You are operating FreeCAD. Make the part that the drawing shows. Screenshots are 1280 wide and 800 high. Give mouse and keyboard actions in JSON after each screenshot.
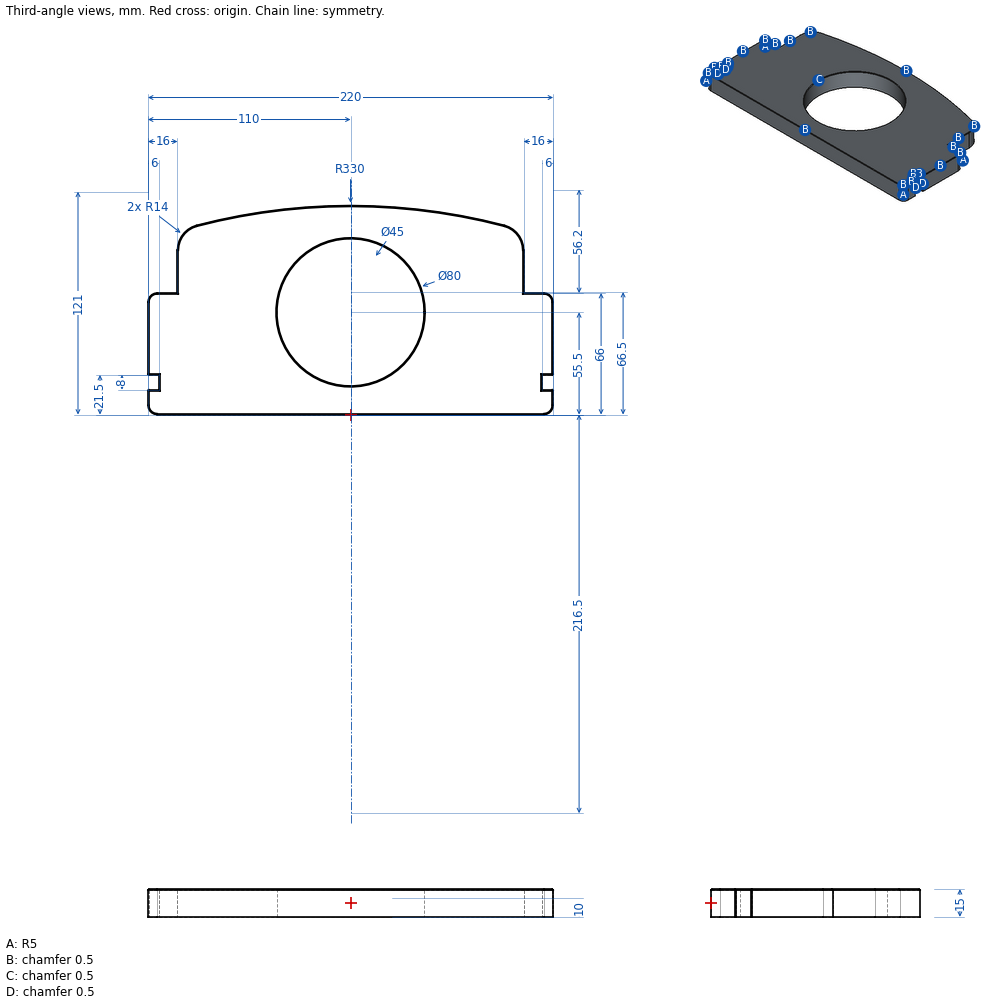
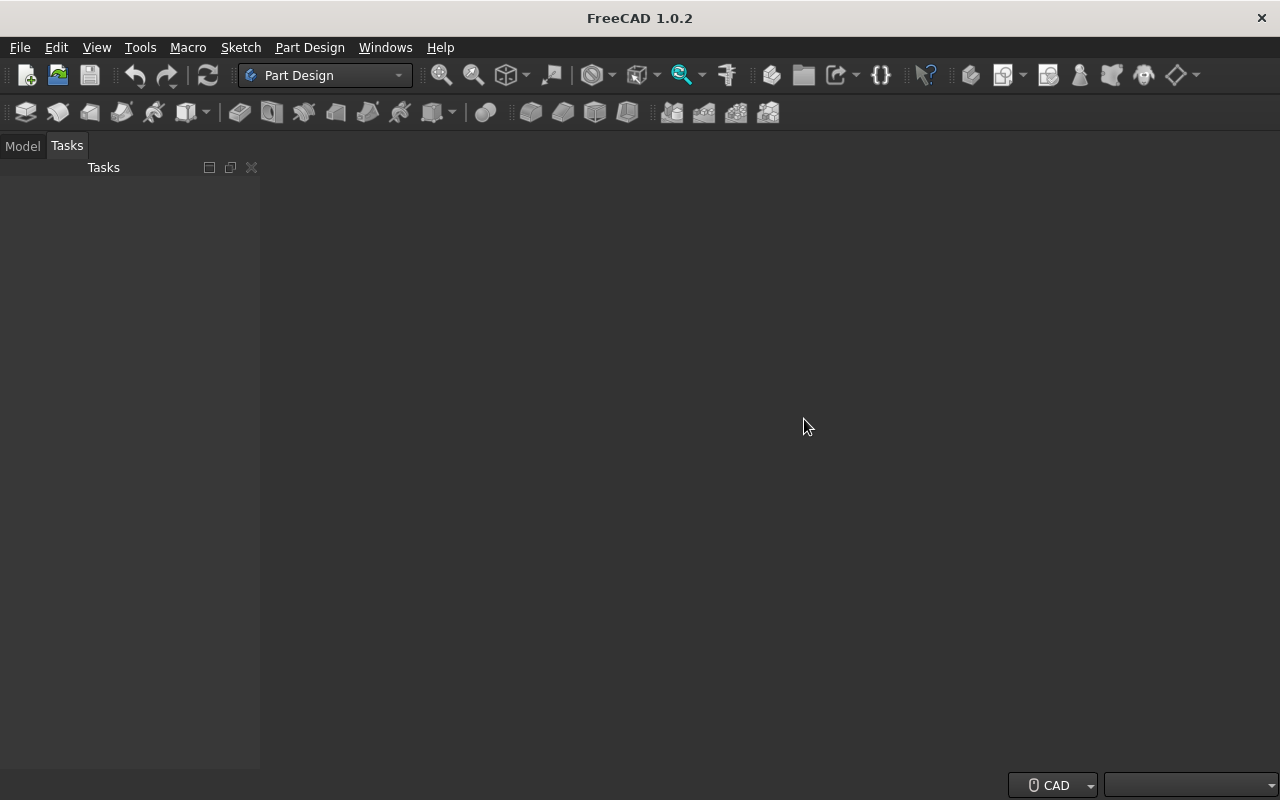
{"action": "left_click", "coordinate": [26, 76]}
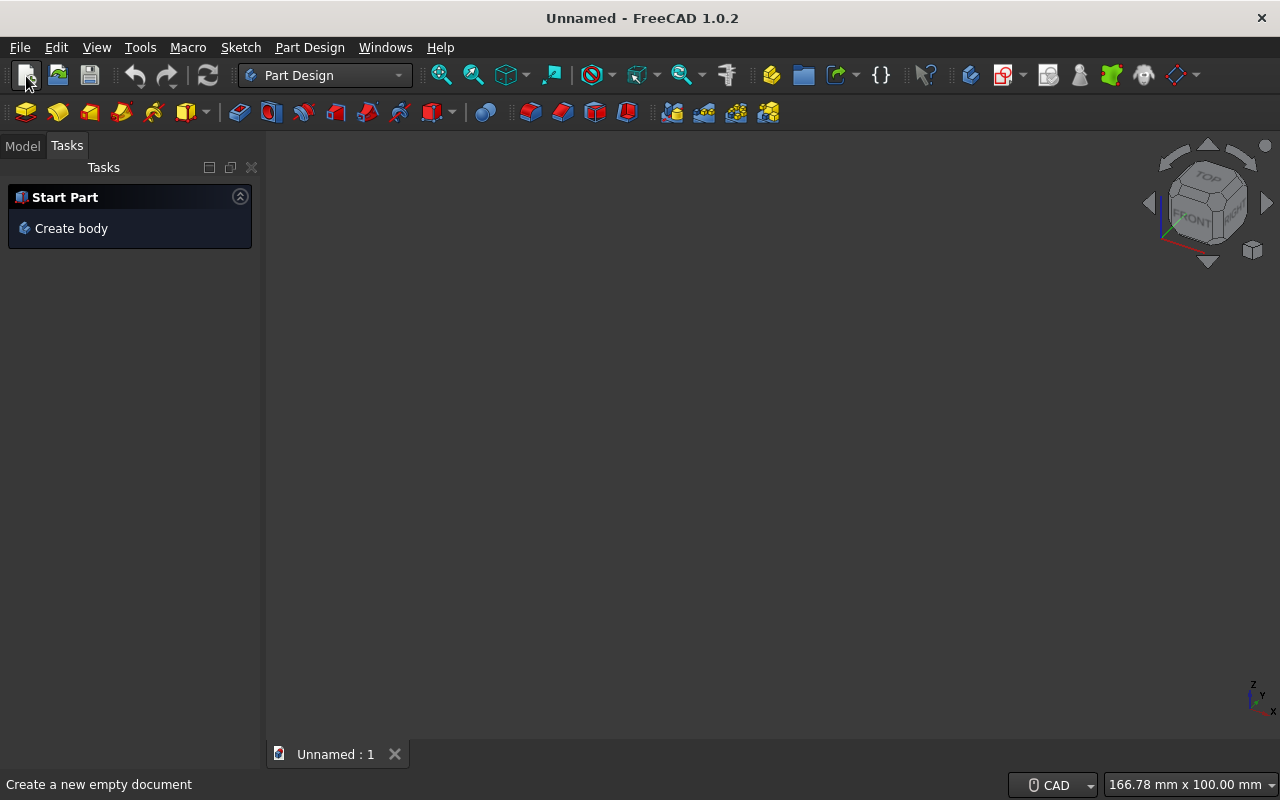
{"action": "left_click", "coordinate": [1004, 76]}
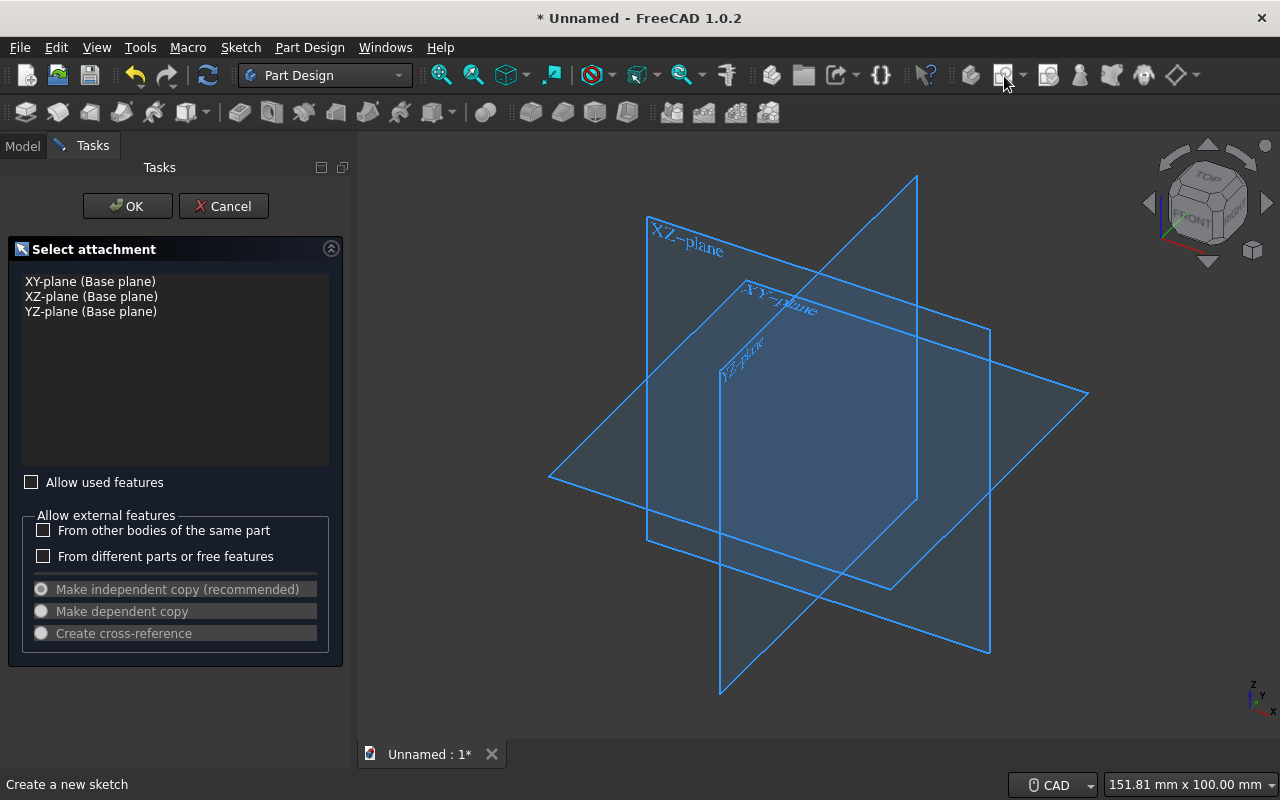
{"action": "left_click", "coordinate": [82, 282]}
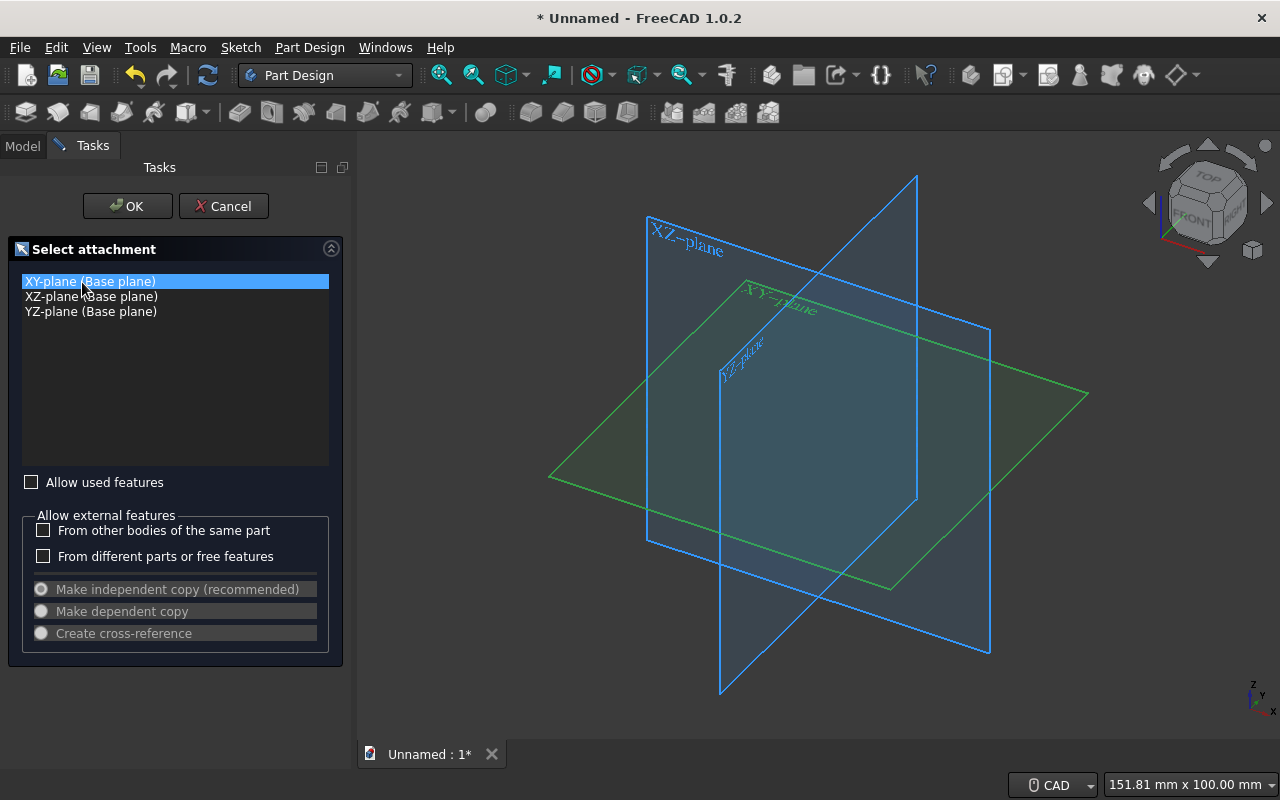
{"action": "left_click", "coordinate": [128, 206]}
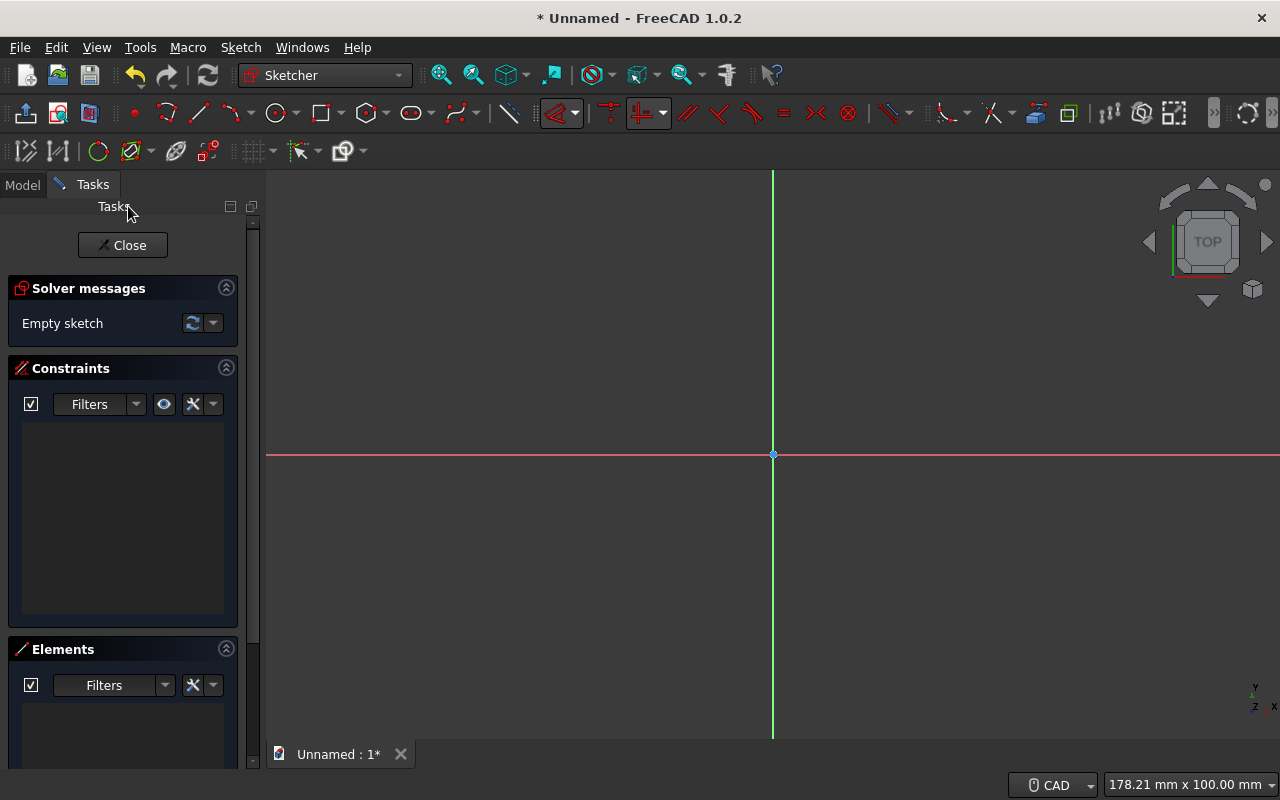
{"action": "scroll", "coordinate": [649, 711], "scroll_direction": "down", "scroll_amount": 4}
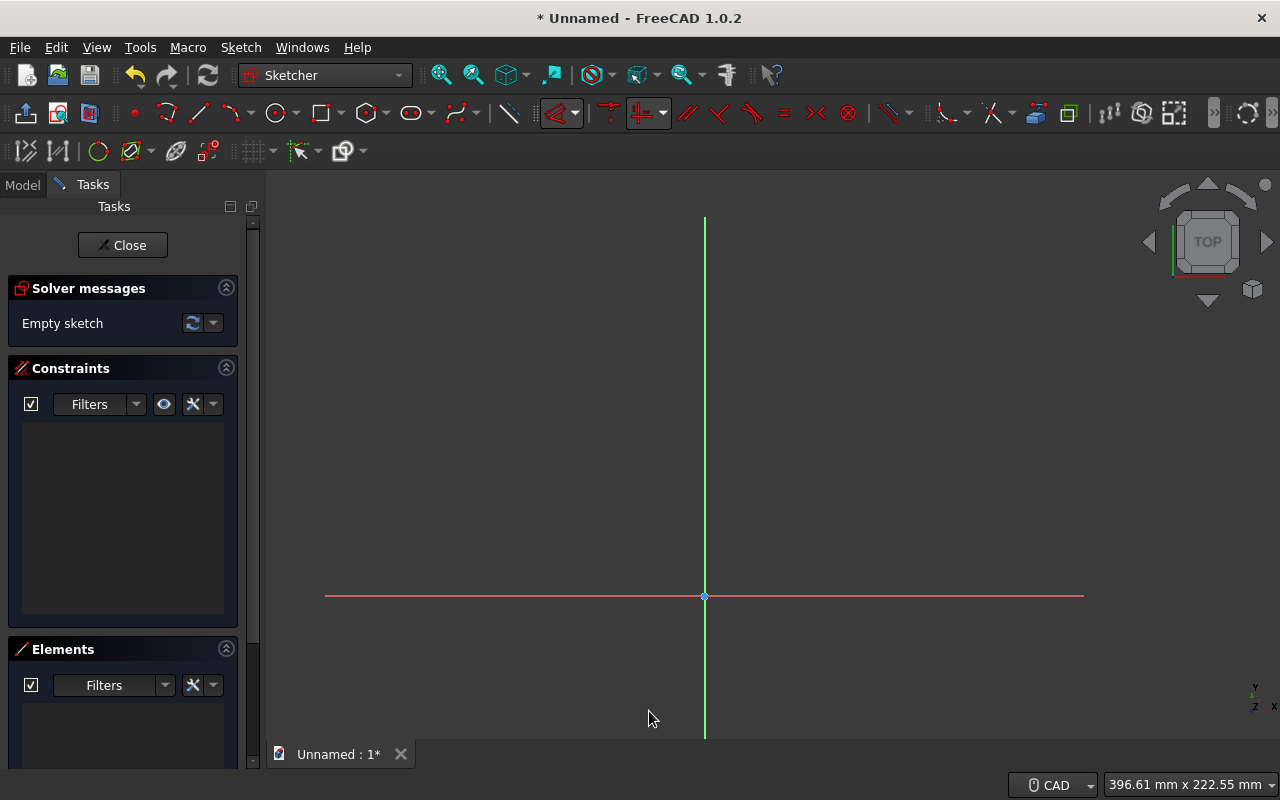
{"action": "left_click", "coordinate": [322, 114]}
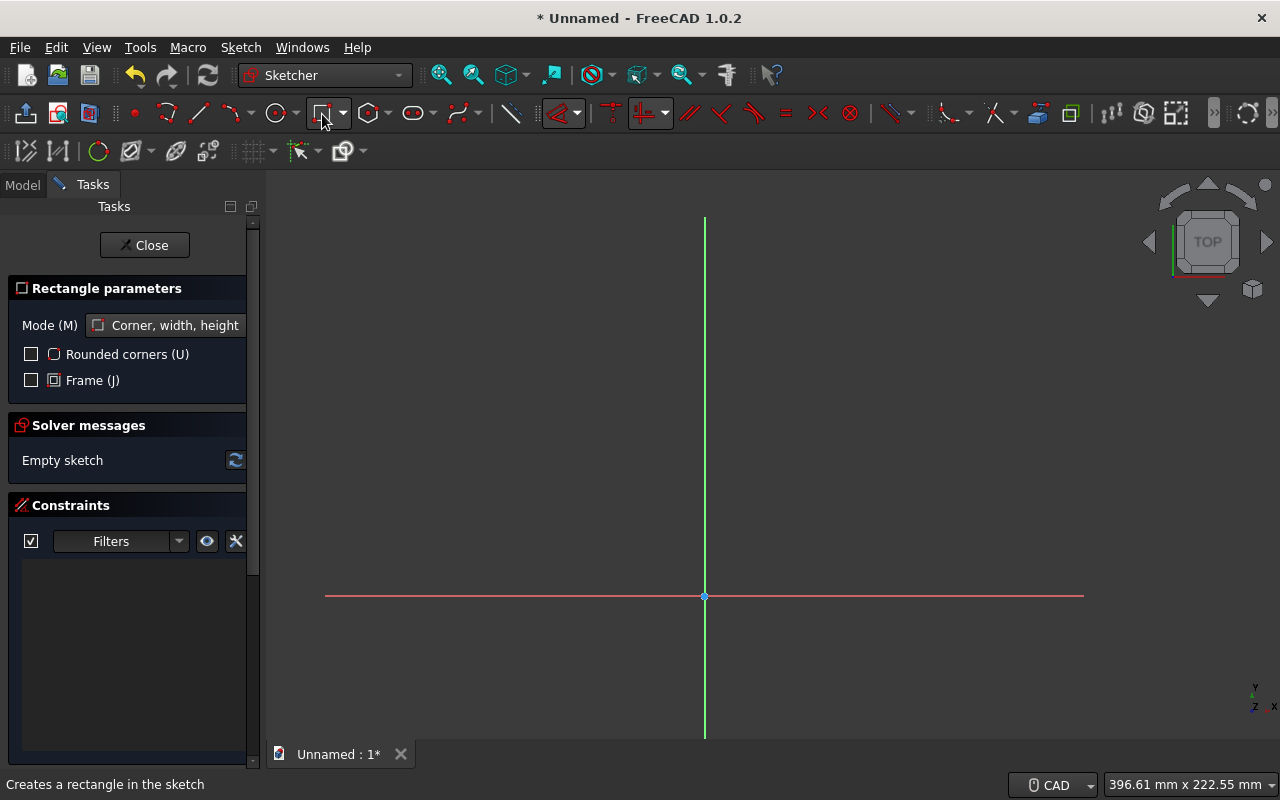
{"action": "left_click", "coordinate": [424, 287]}
{"action": "left_click", "coordinate": [986, 596]}
{"action": "key", "text": "Escape"}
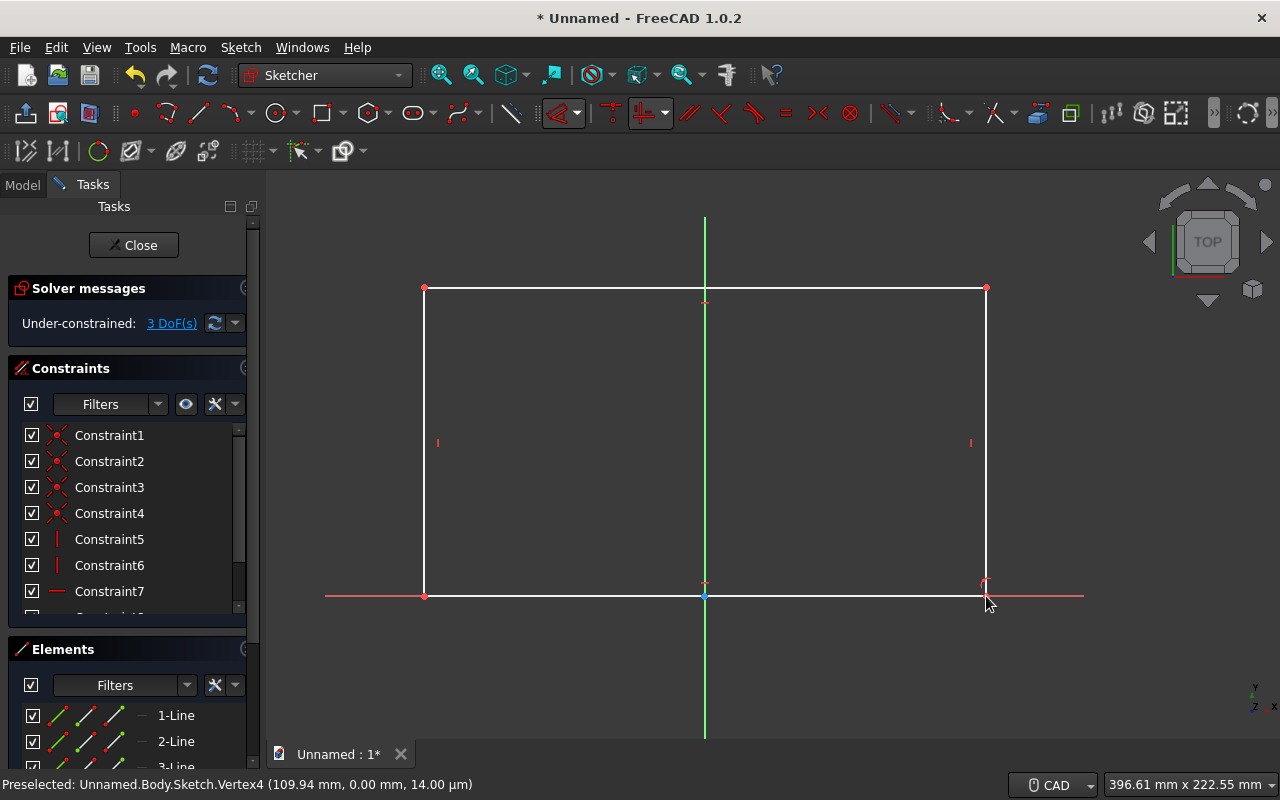
{"action": "left_click", "coordinate": [558, 114]}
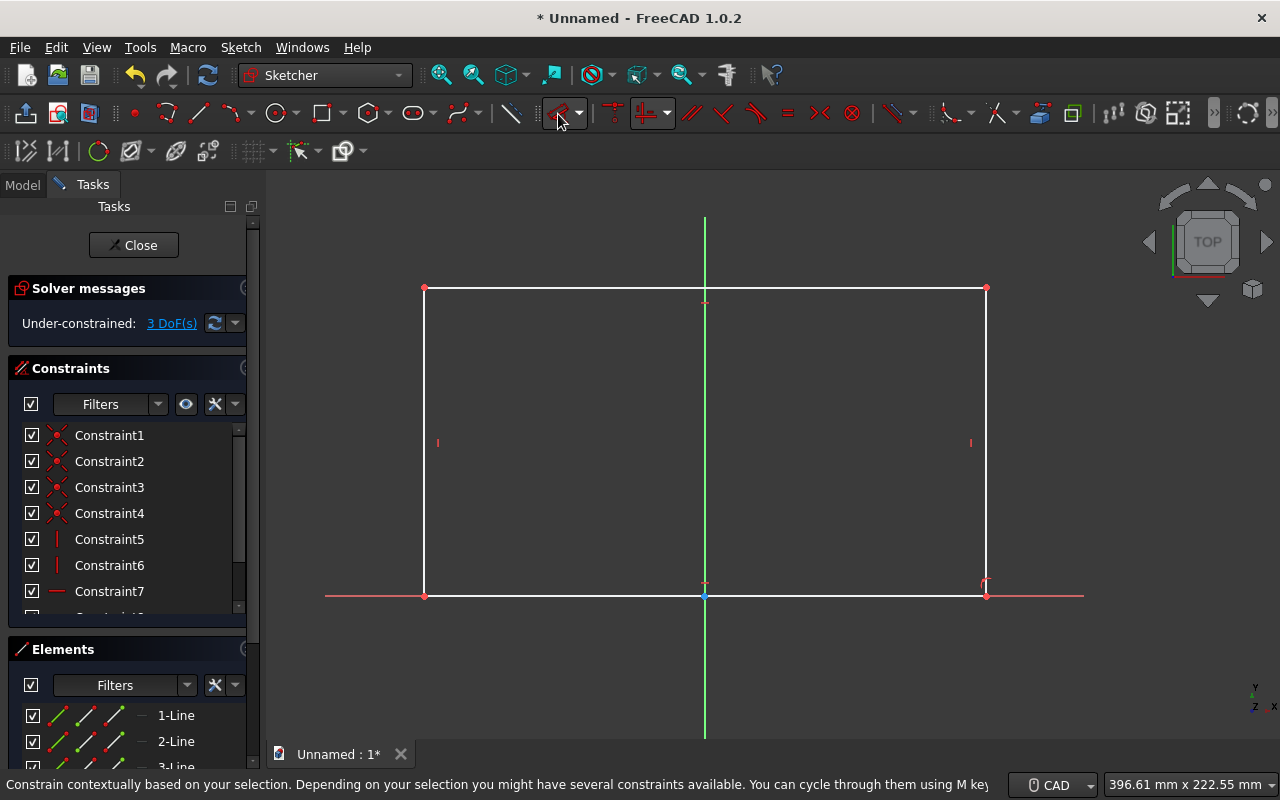
{"action": "left_click", "coordinate": [424, 380]}
{"action": "left_click", "coordinate": [390, 442]}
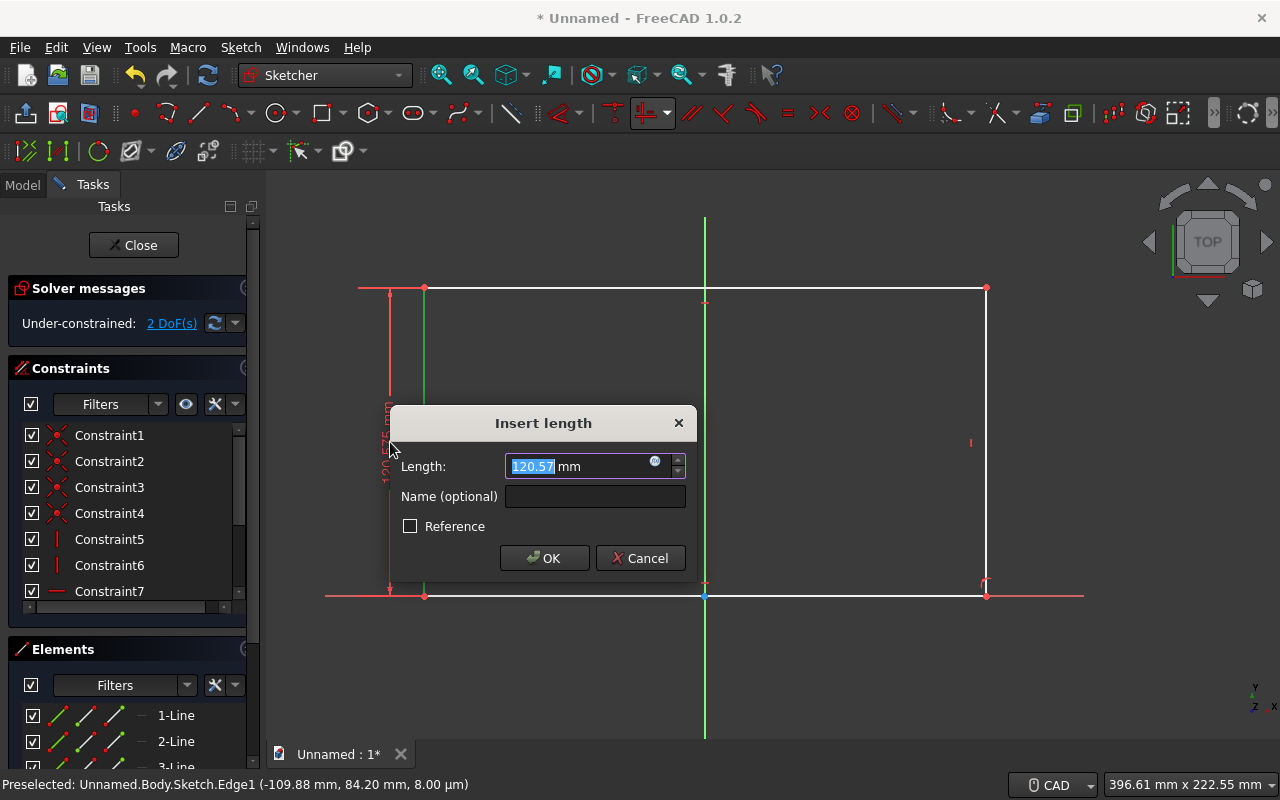
{"action": "type", "text": "121"}
{"action": "key", "text": "Return"}